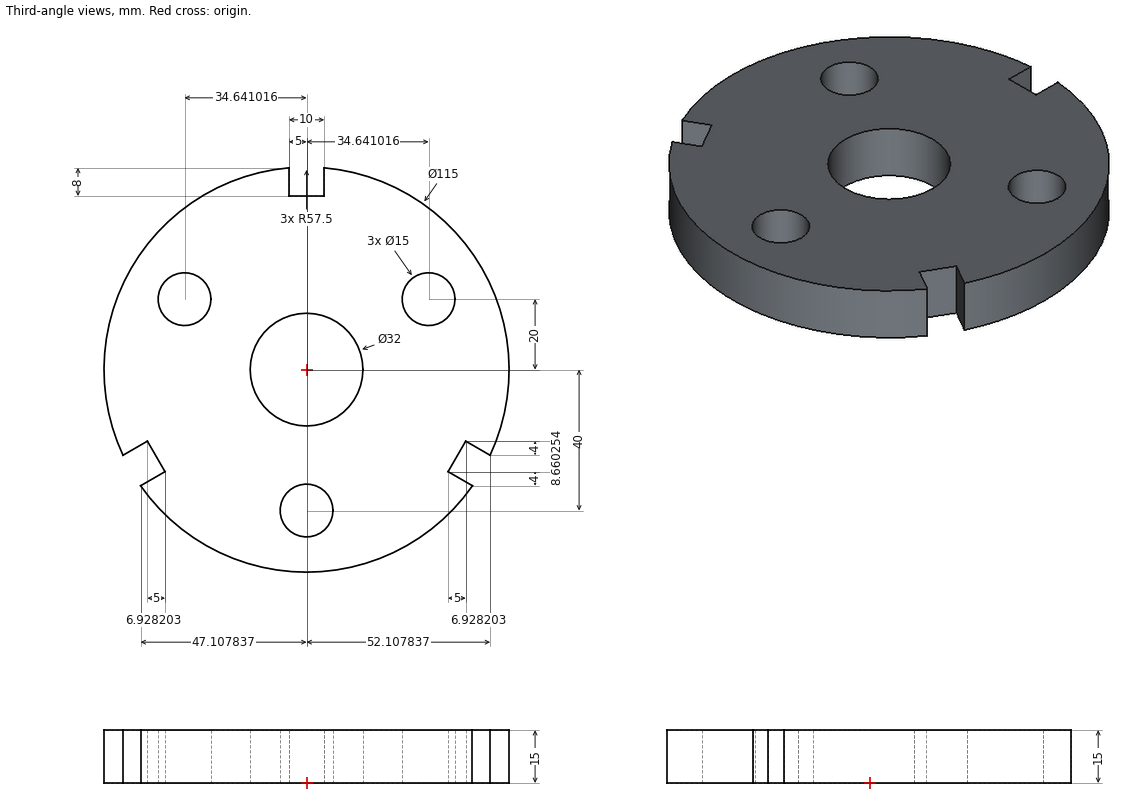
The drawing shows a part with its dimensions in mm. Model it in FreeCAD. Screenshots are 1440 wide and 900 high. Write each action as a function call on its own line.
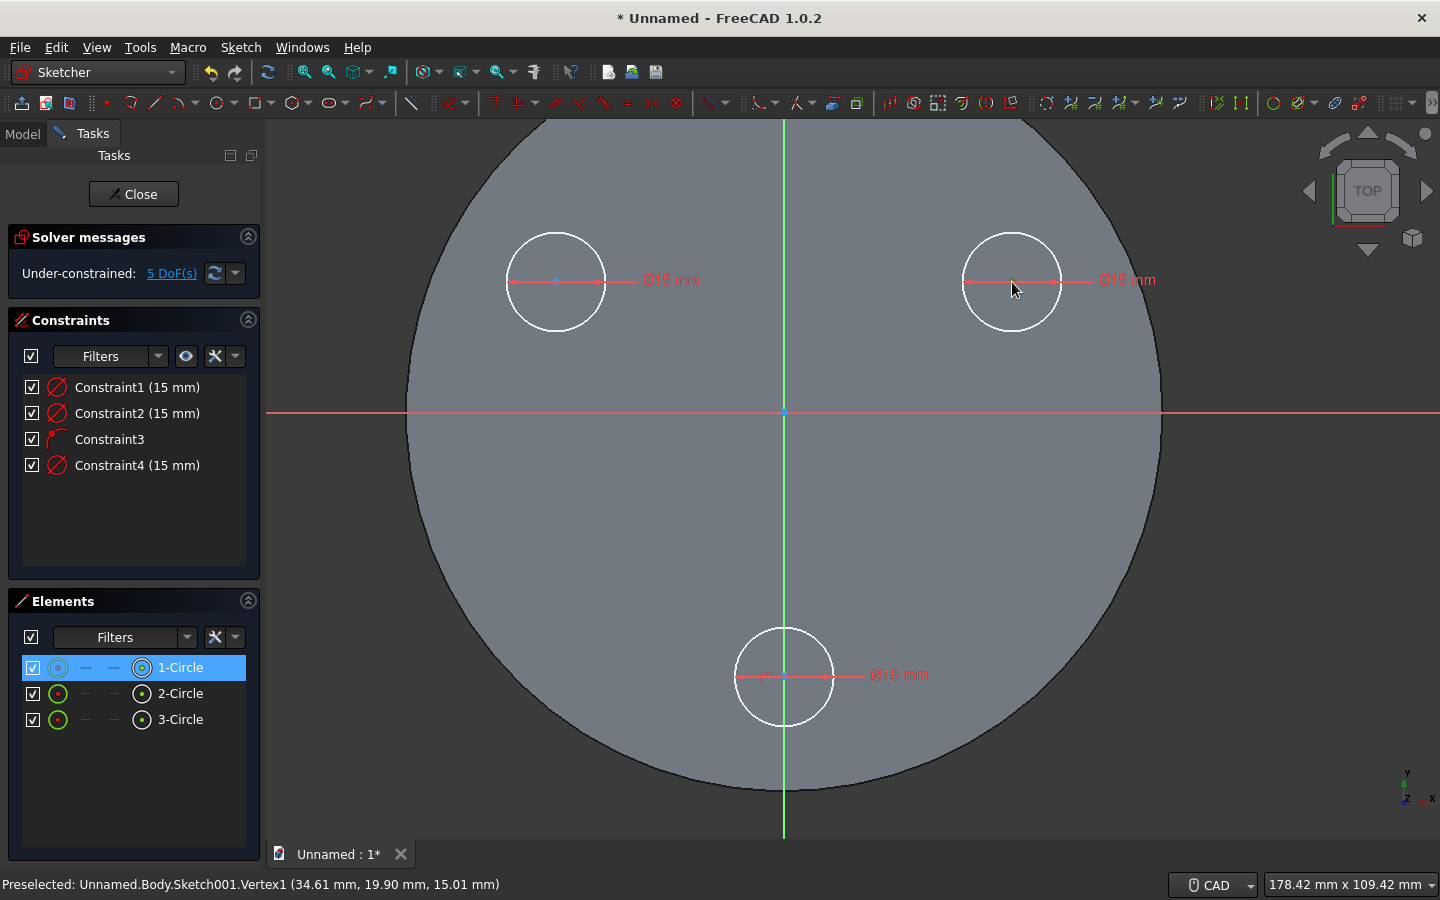
click(556, 282)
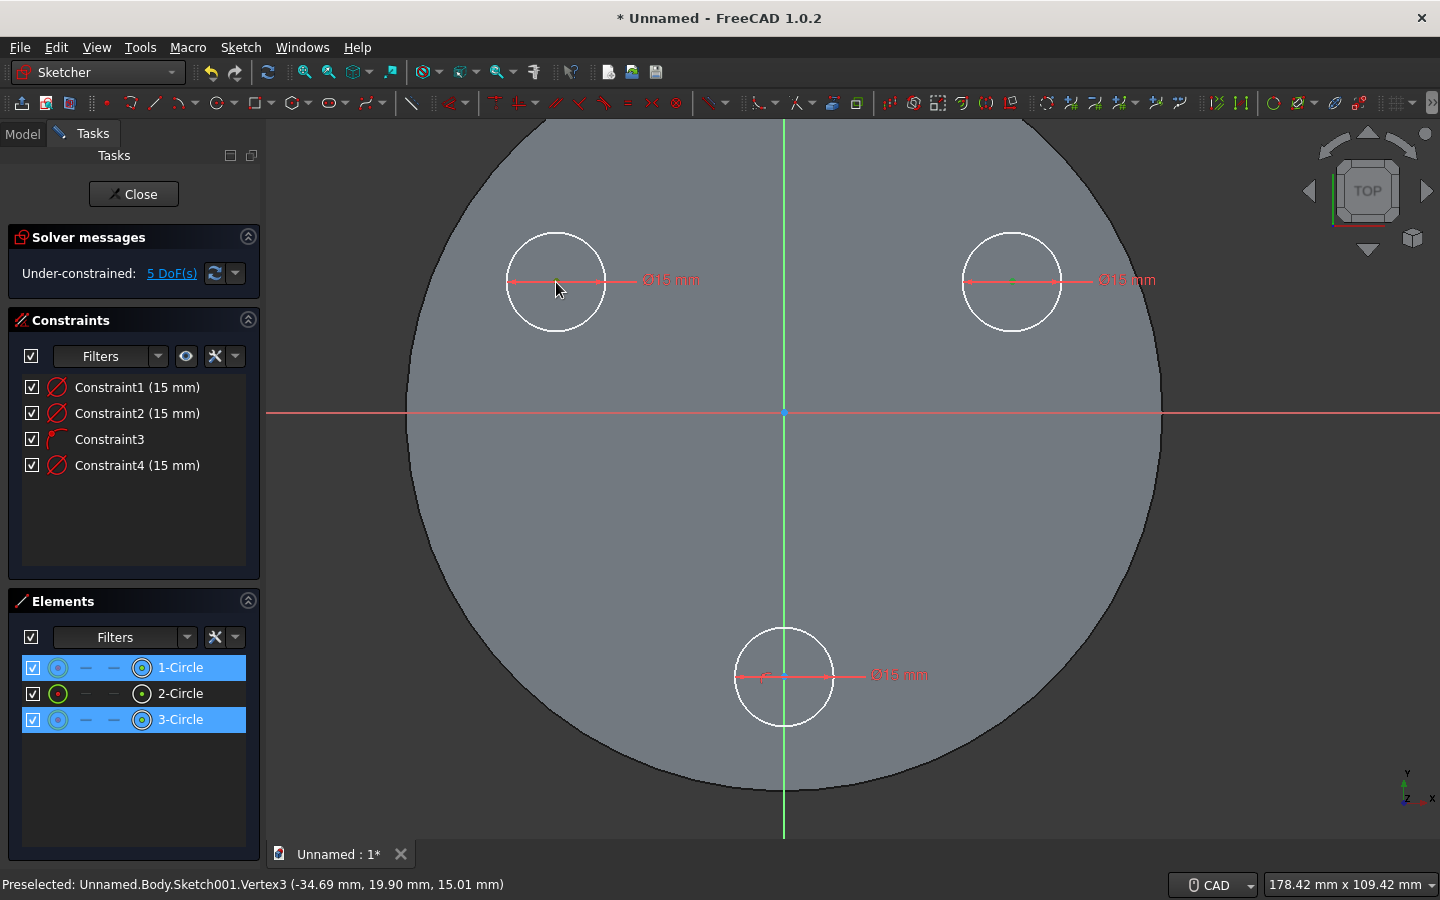
key(h)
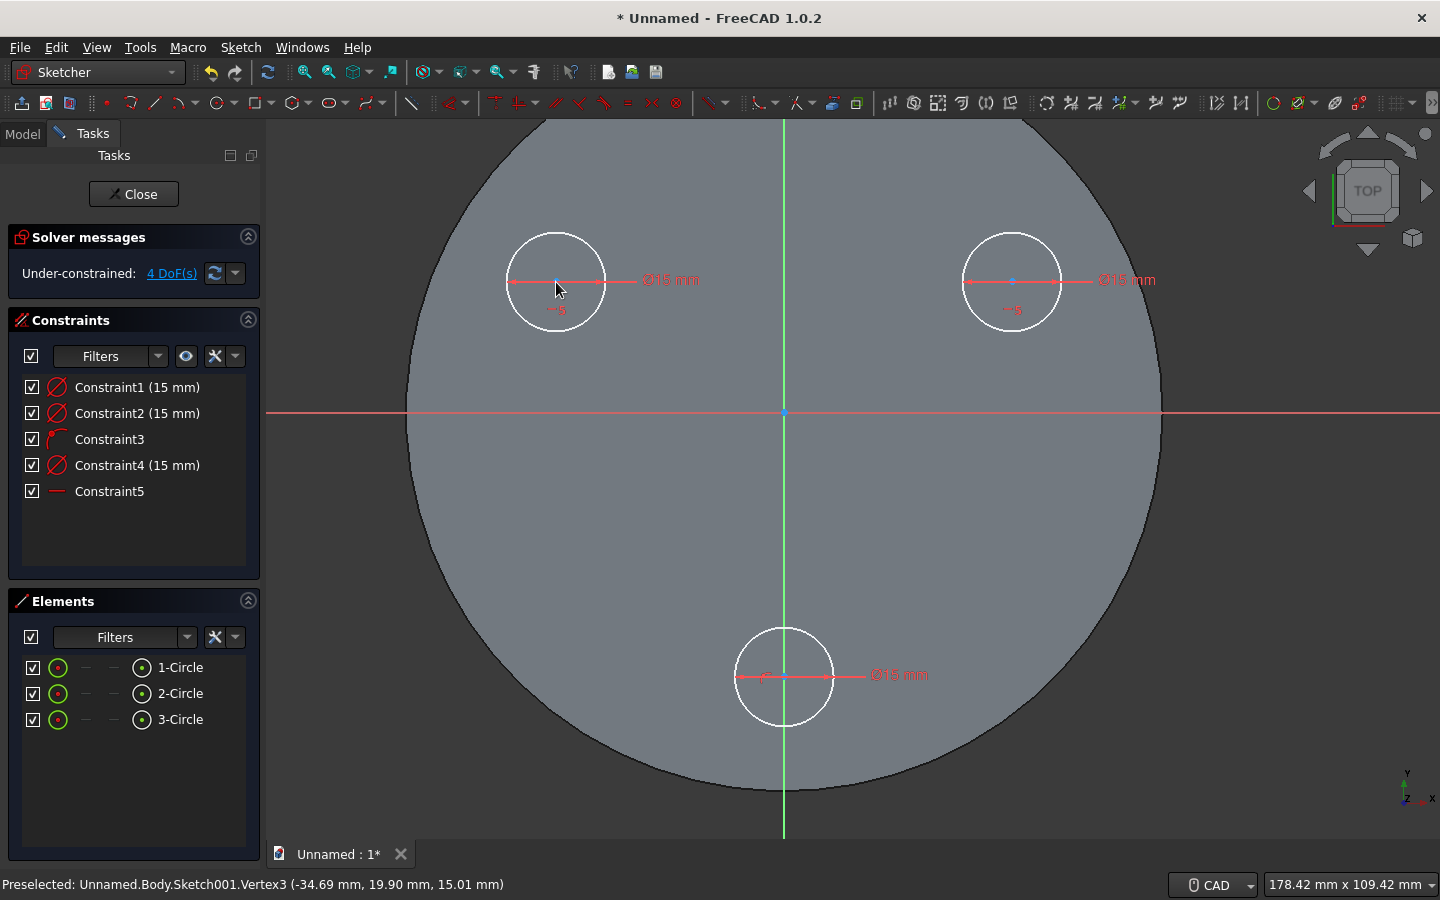
key(d)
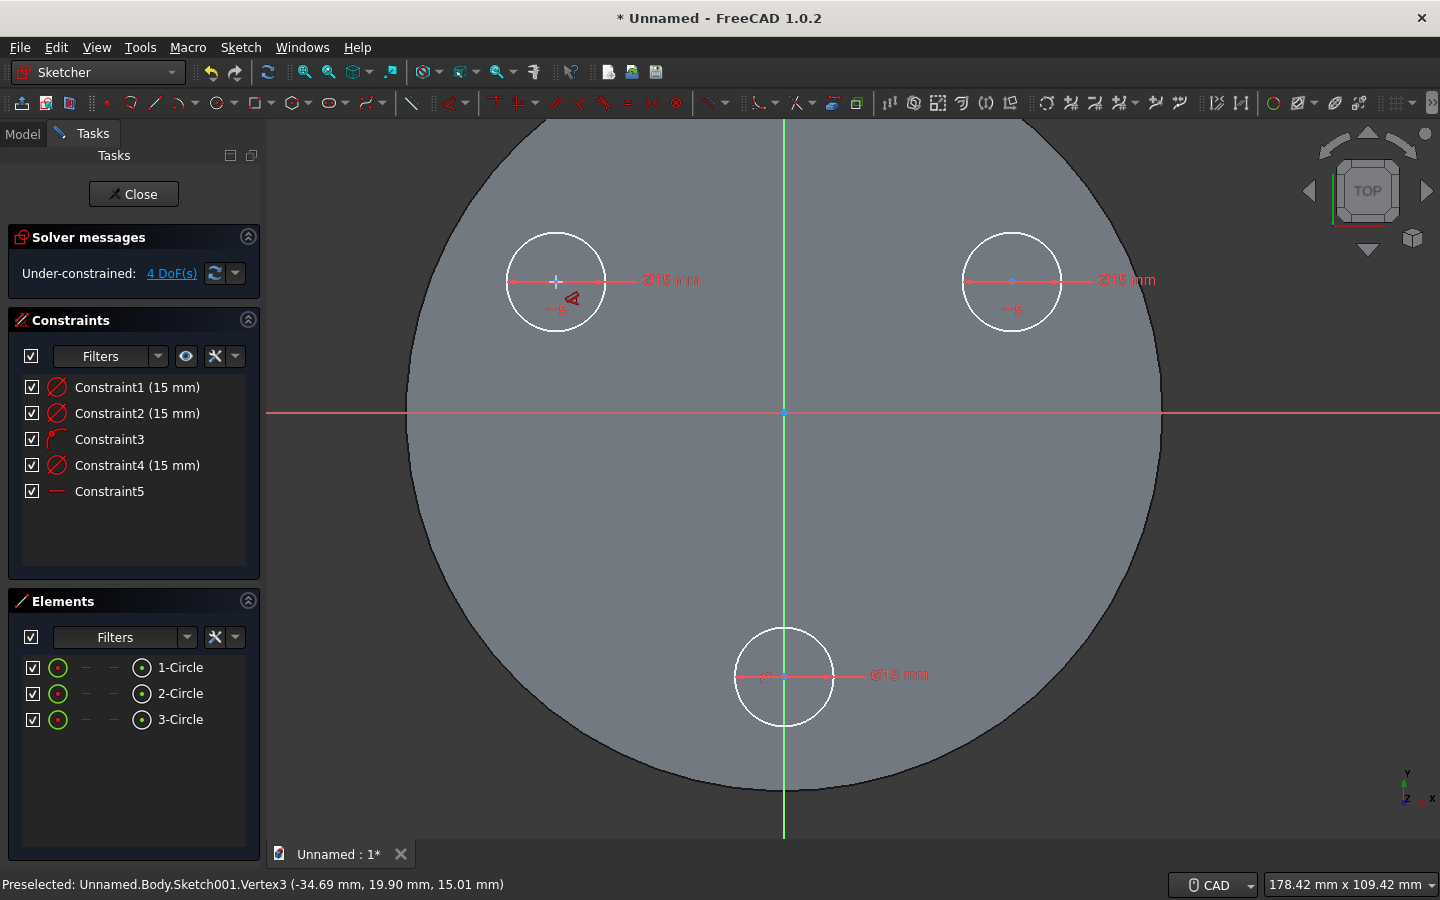
click(1012, 282)
click(1046, 347)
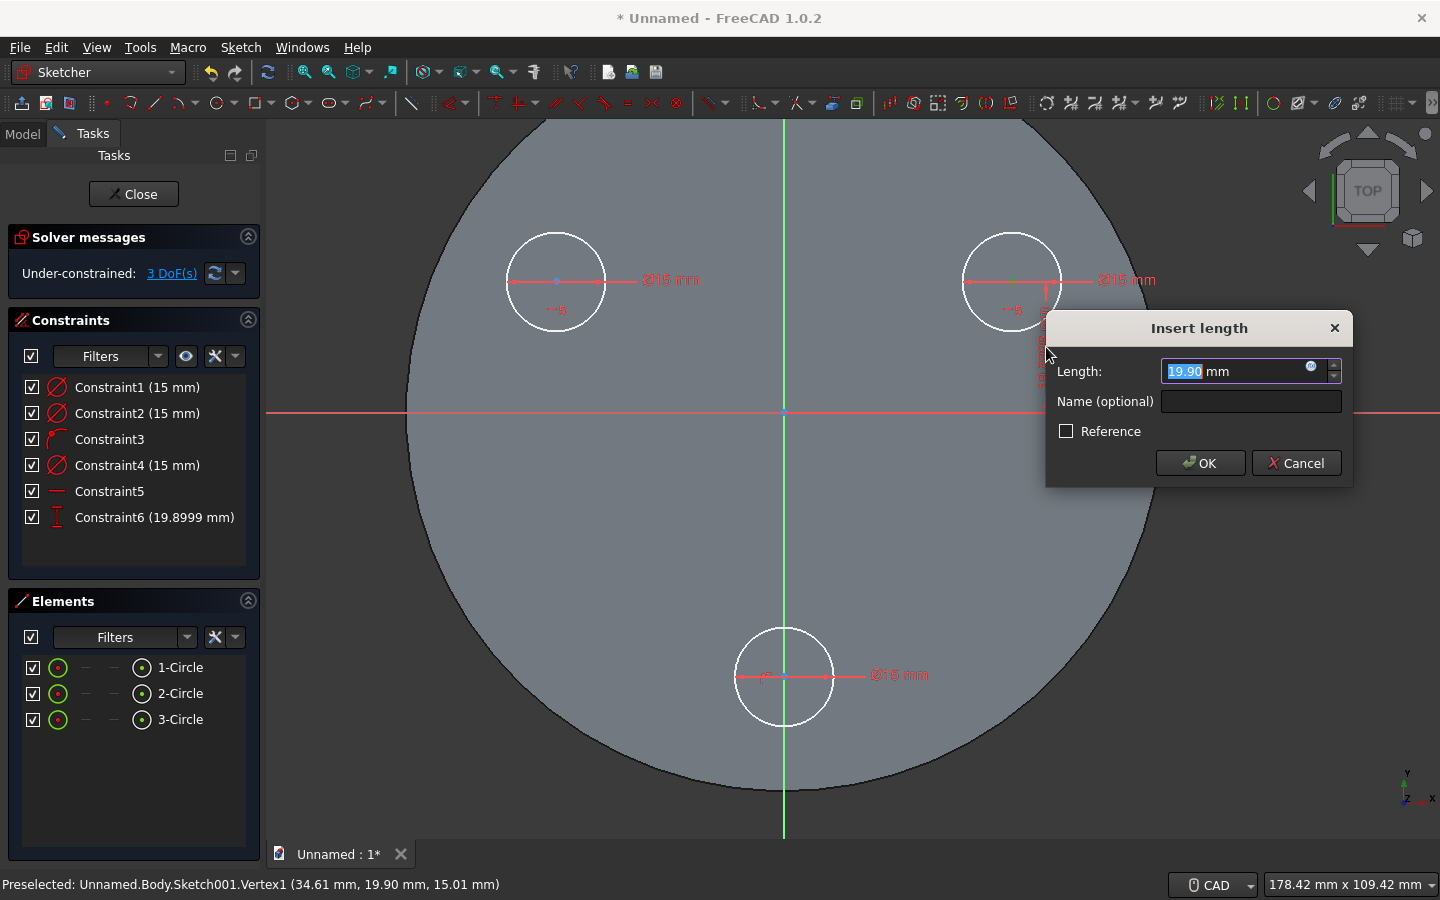
text(20)
key(Return)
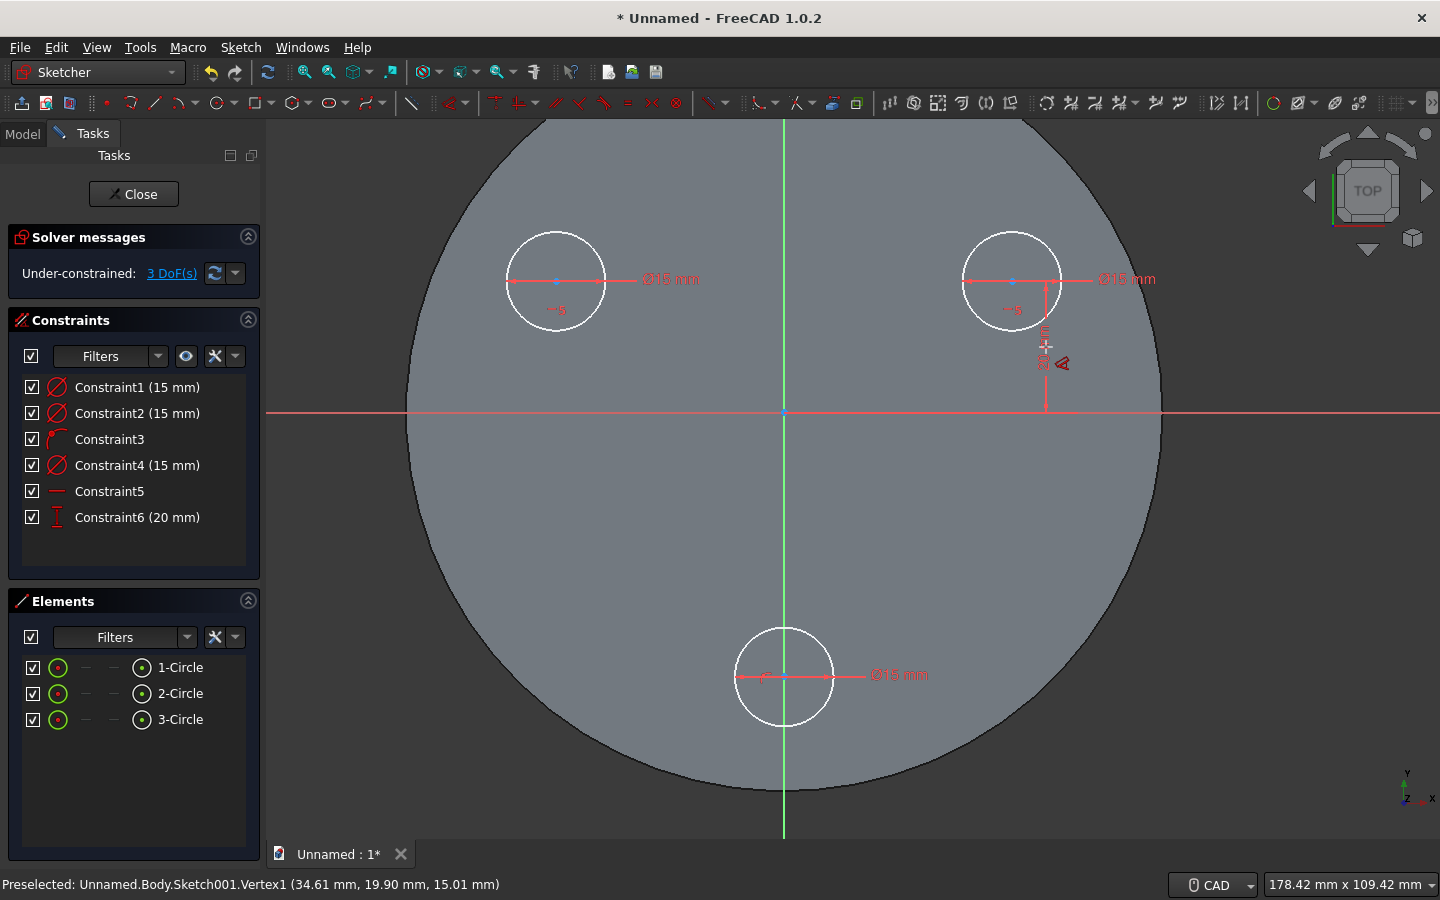
click(784, 677)
click(818, 545)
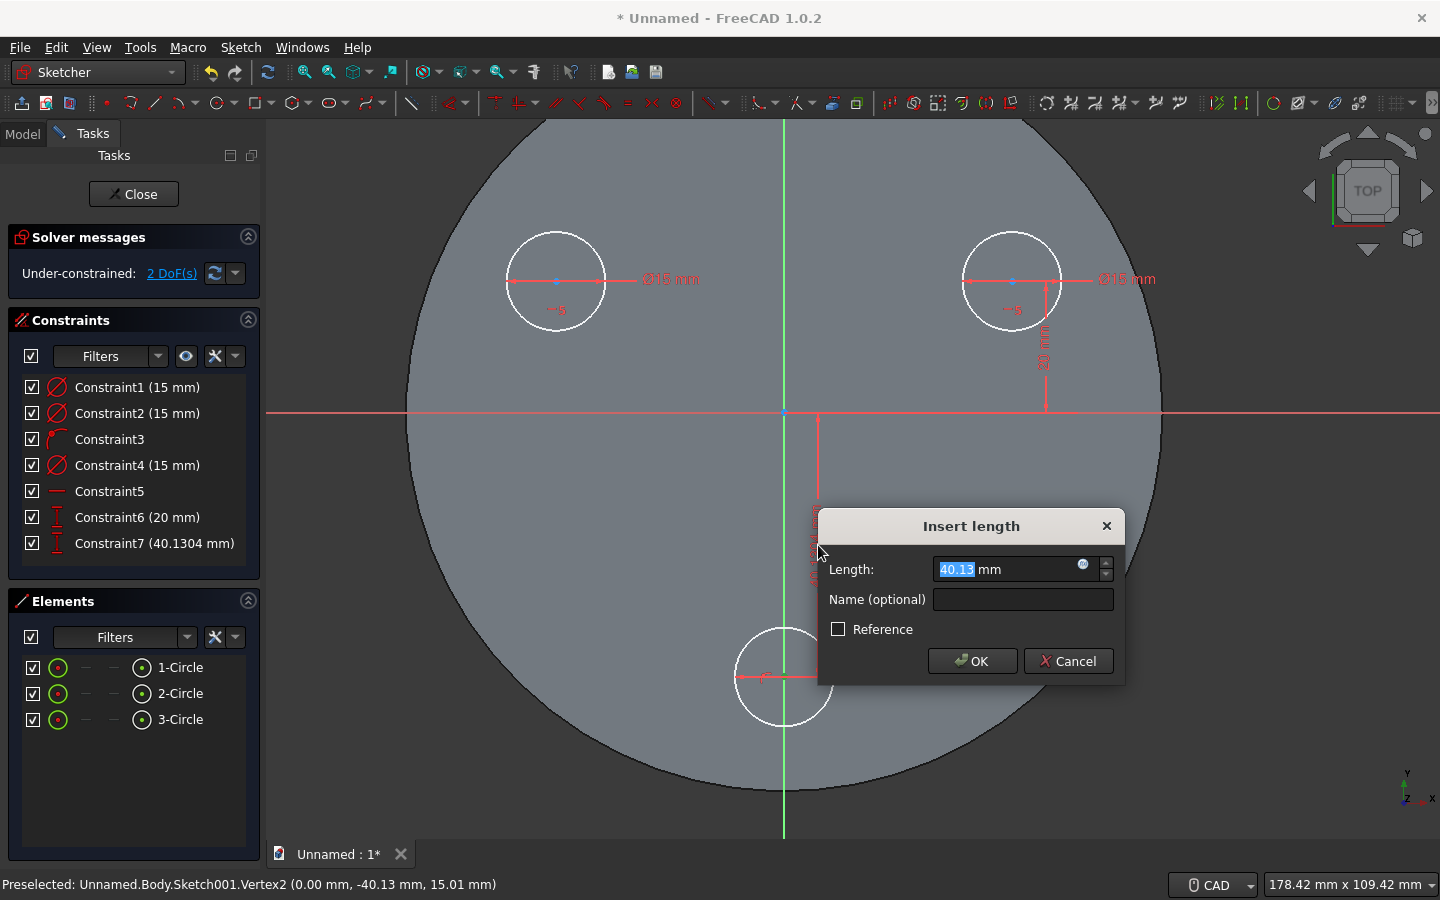
text(40)
key(Return)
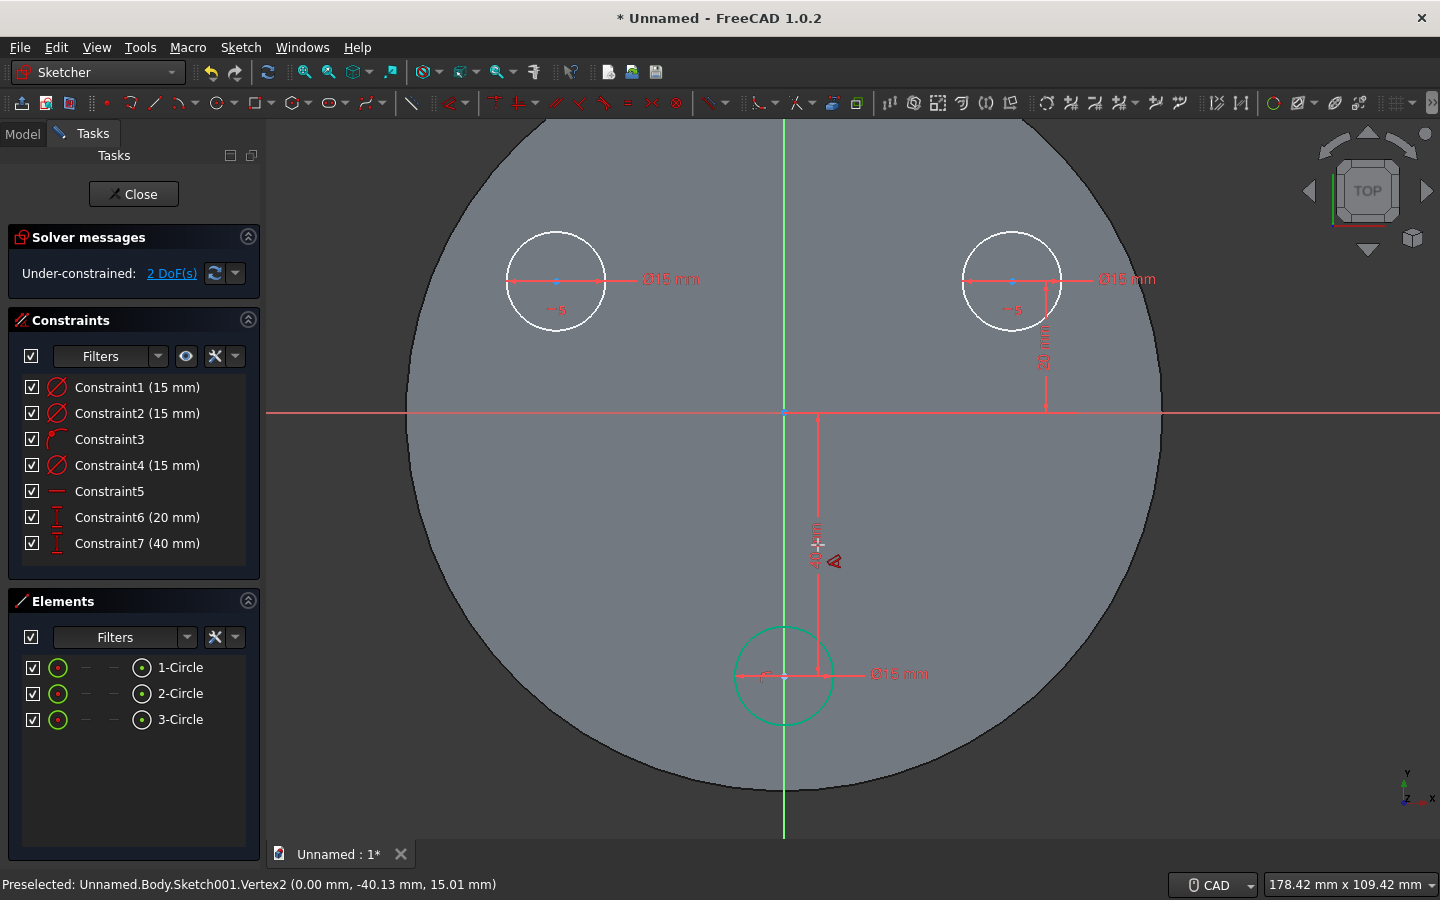
click(1012, 281)
click(898, 247)